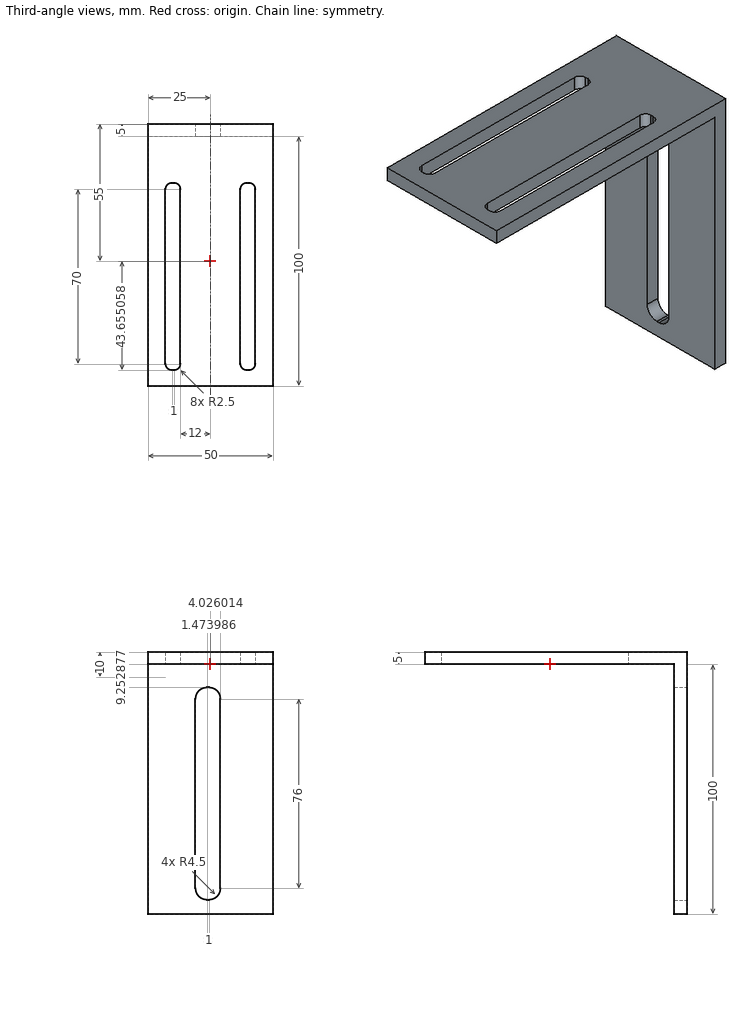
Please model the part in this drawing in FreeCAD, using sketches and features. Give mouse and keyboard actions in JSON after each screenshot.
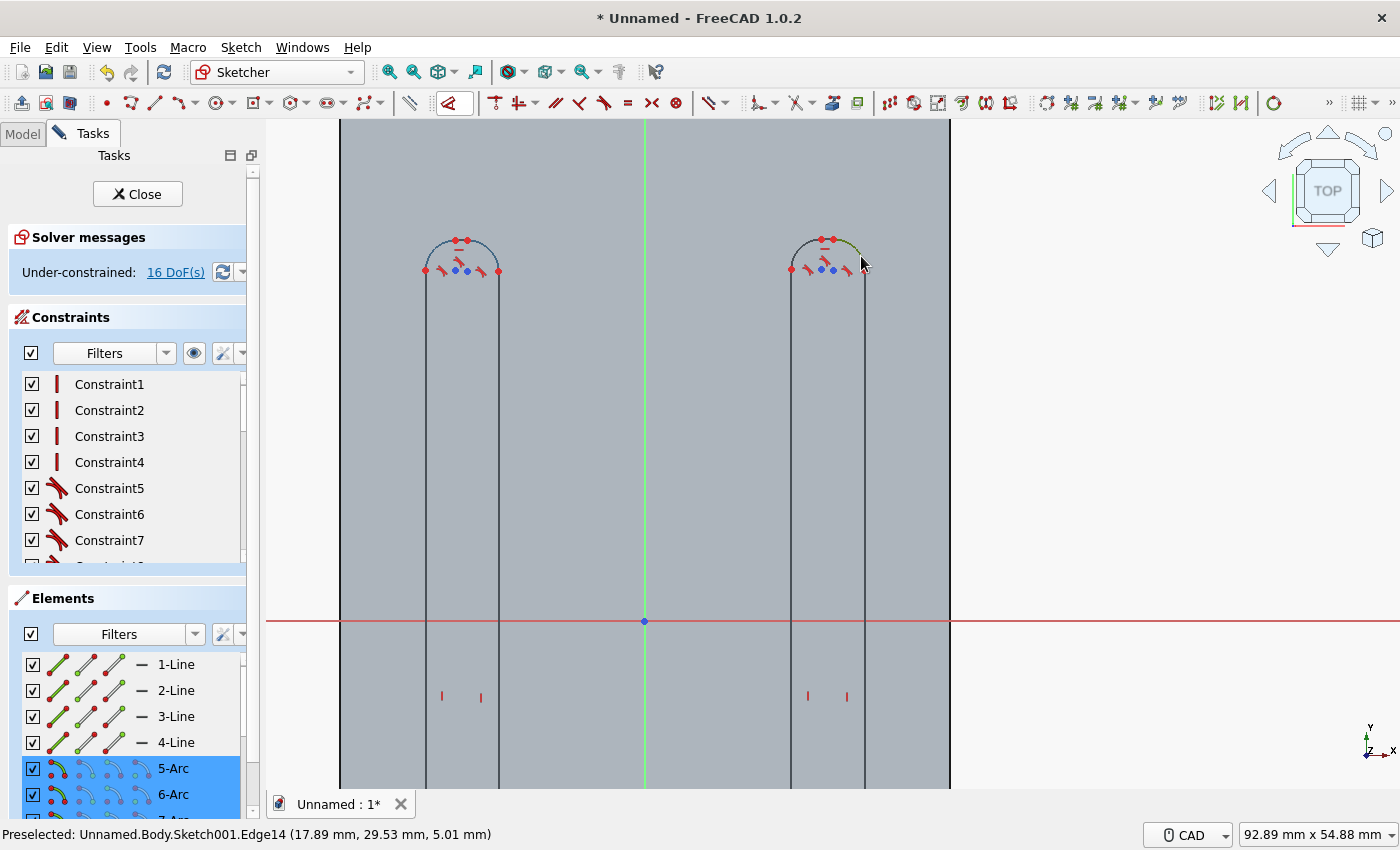
{"action": "left_click", "coordinate": [808, 243]}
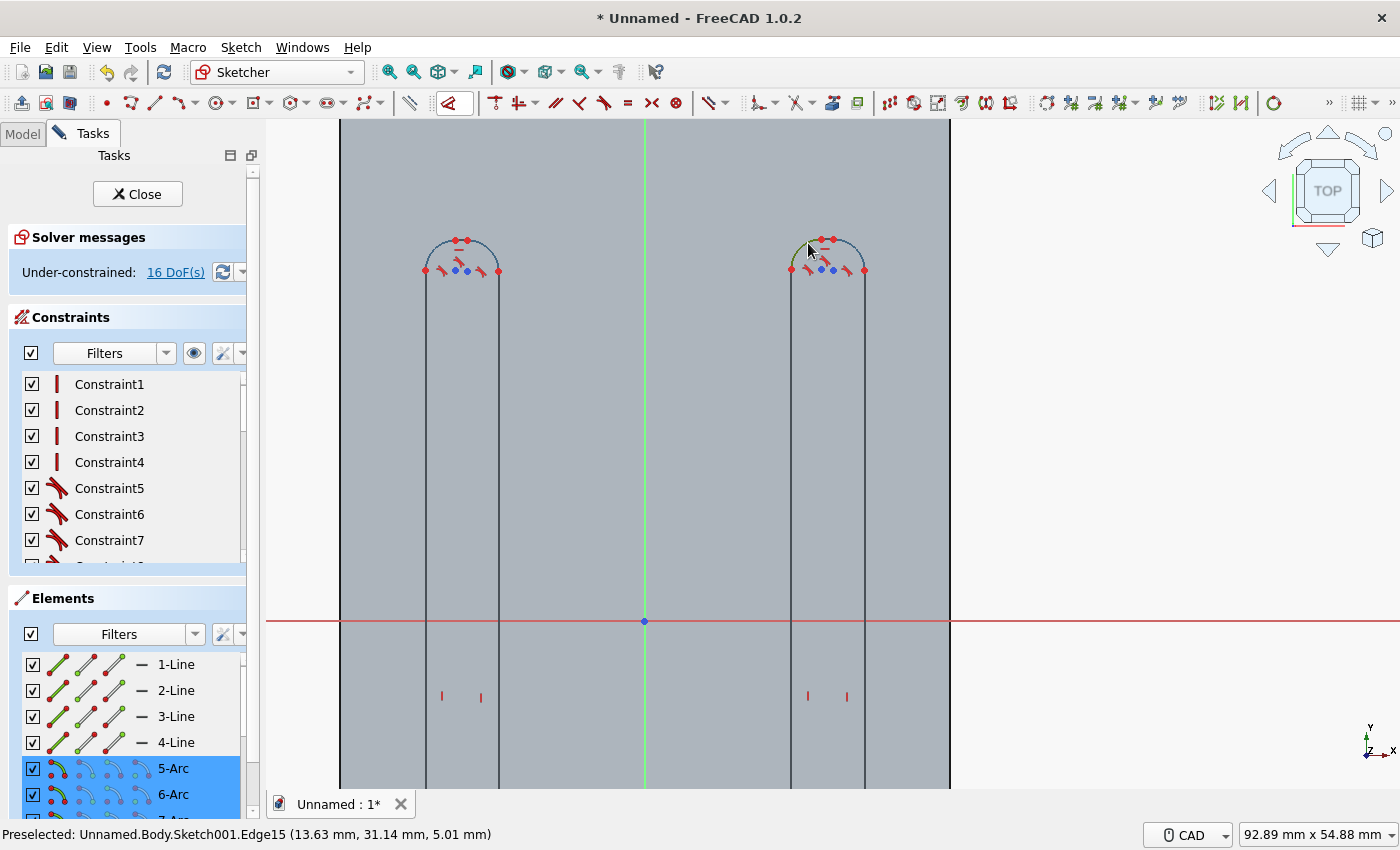
{"action": "scroll", "coordinate": [862, 256], "scroll_direction": "down", "scroll_amount": 4}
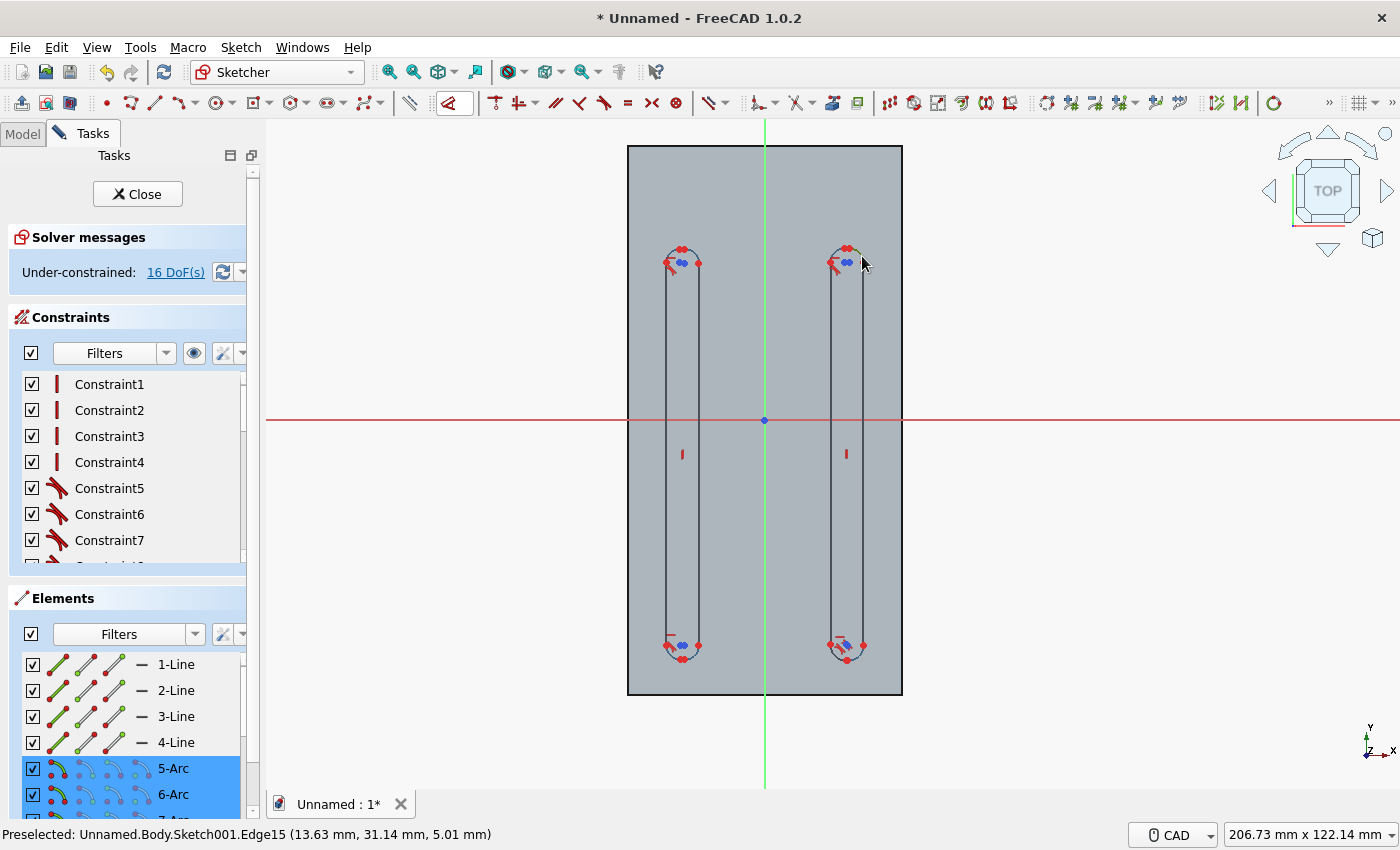
{"action": "scroll", "coordinate": [832, 652], "scroll_direction": "up", "scroll_amount": 4}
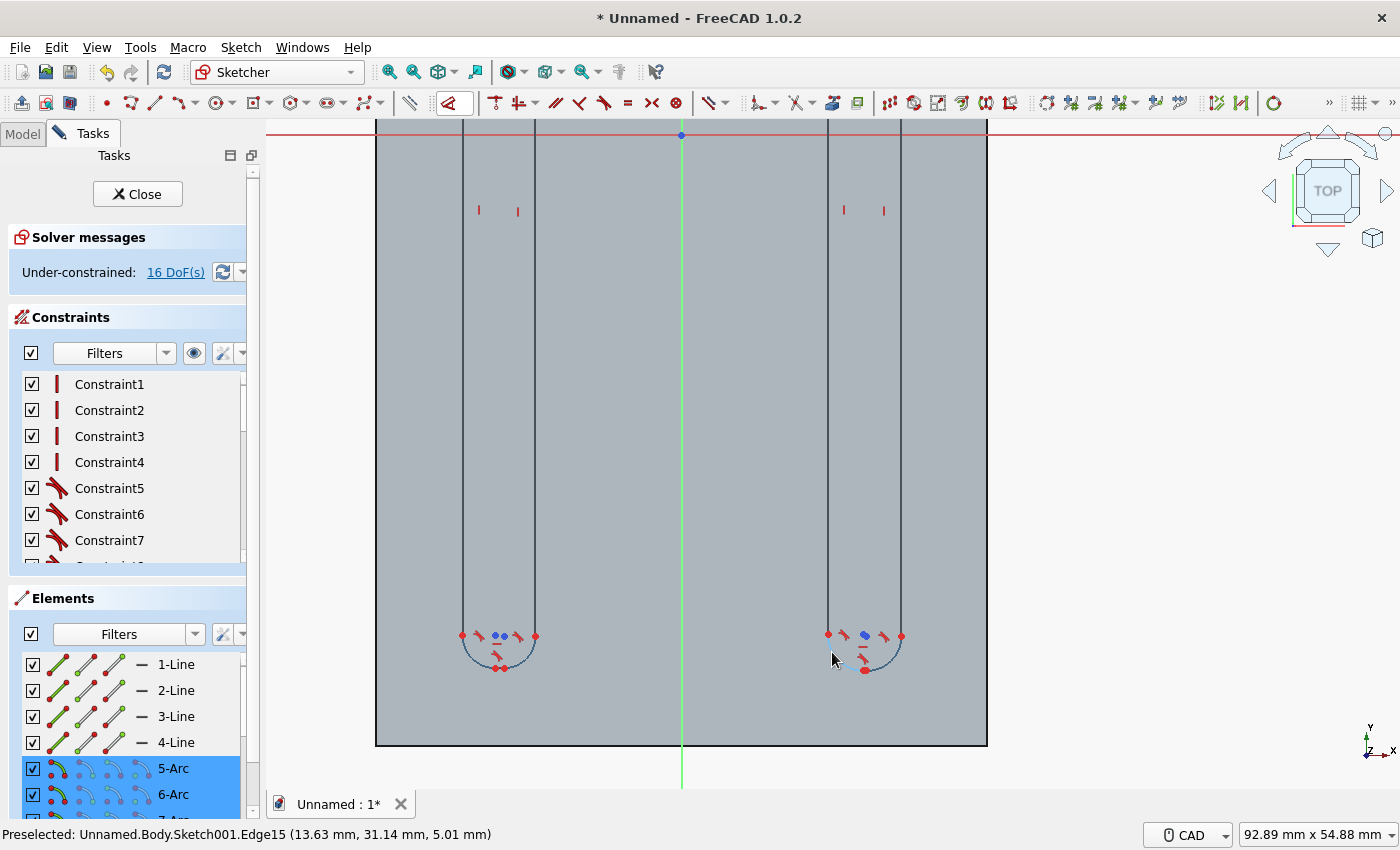
{"action": "left_click", "coordinate": [832, 651]}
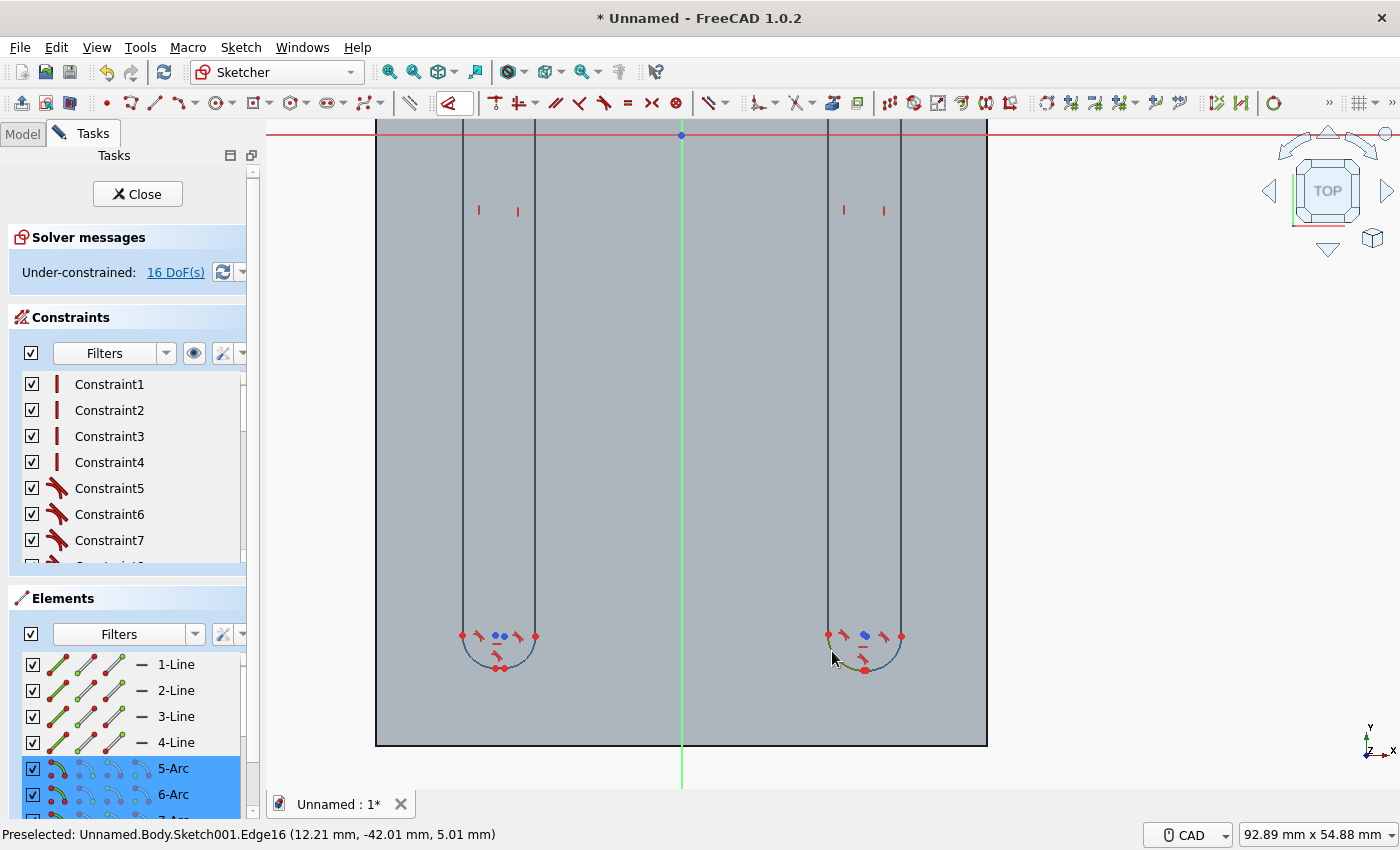
{"action": "left_click", "coordinate": [628, 104]}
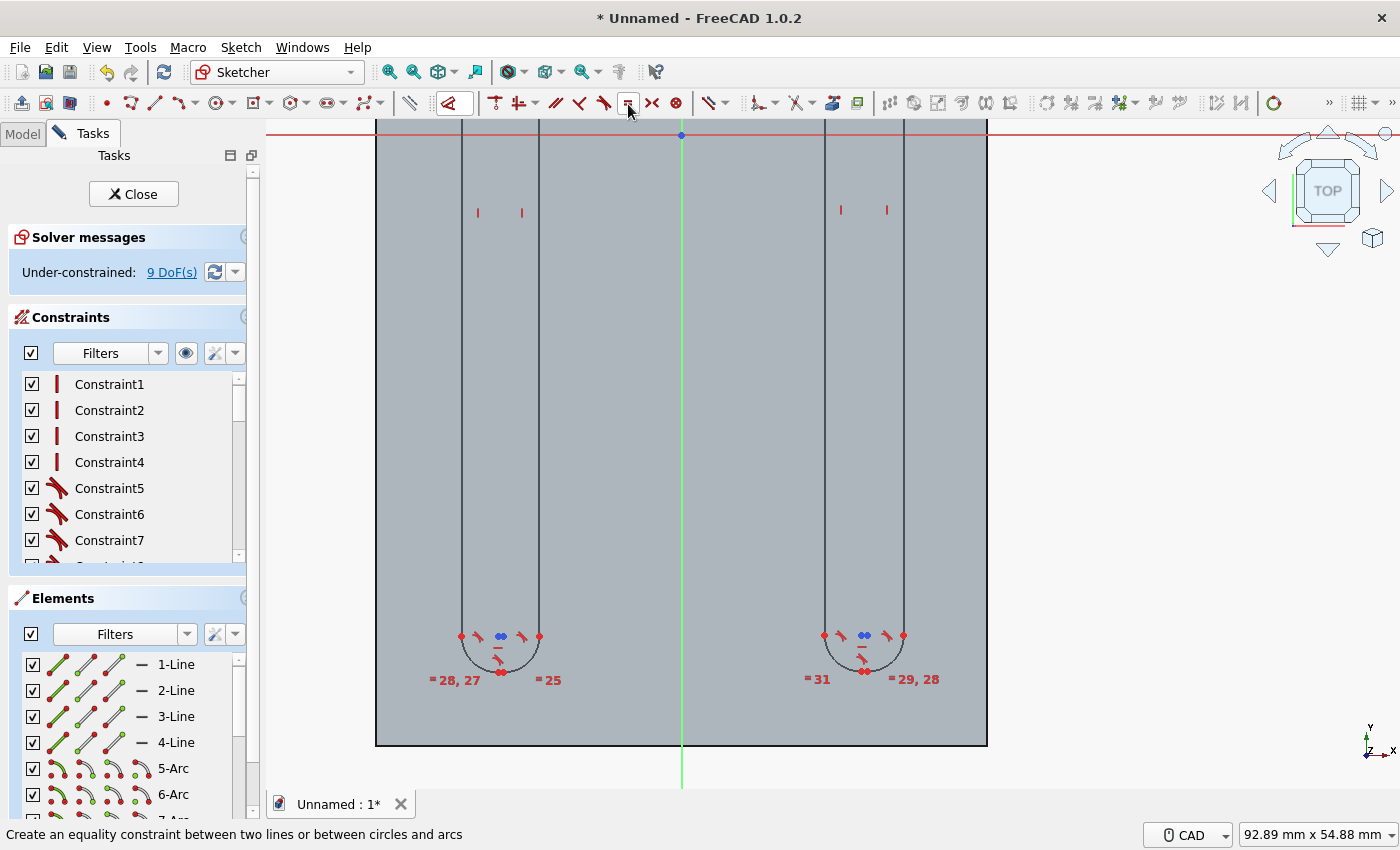
{"action": "scroll", "coordinate": [498, 636], "scroll_direction": "up", "scroll_amount": 5}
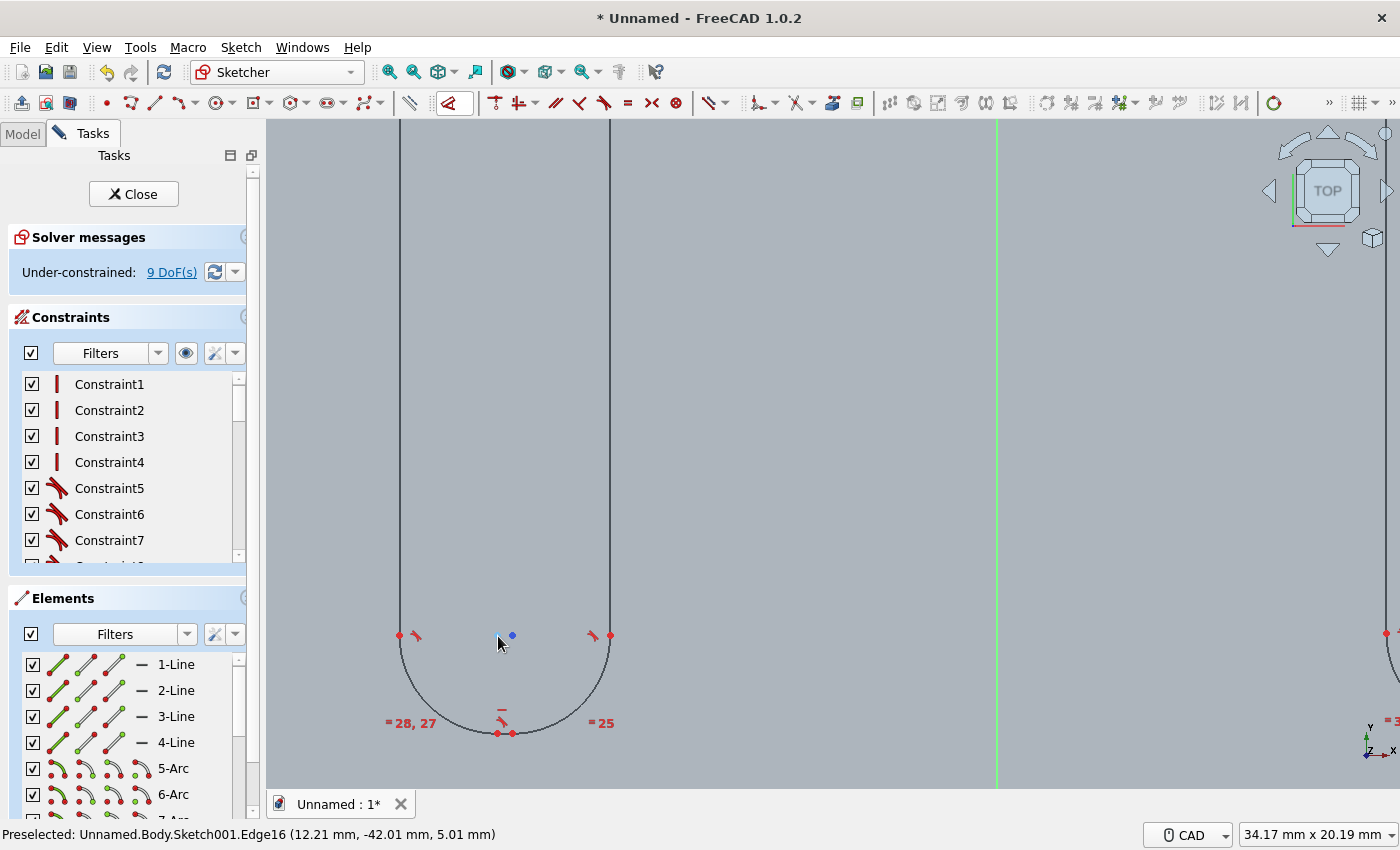
{"action": "left_click", "coordinate": [498, 636]}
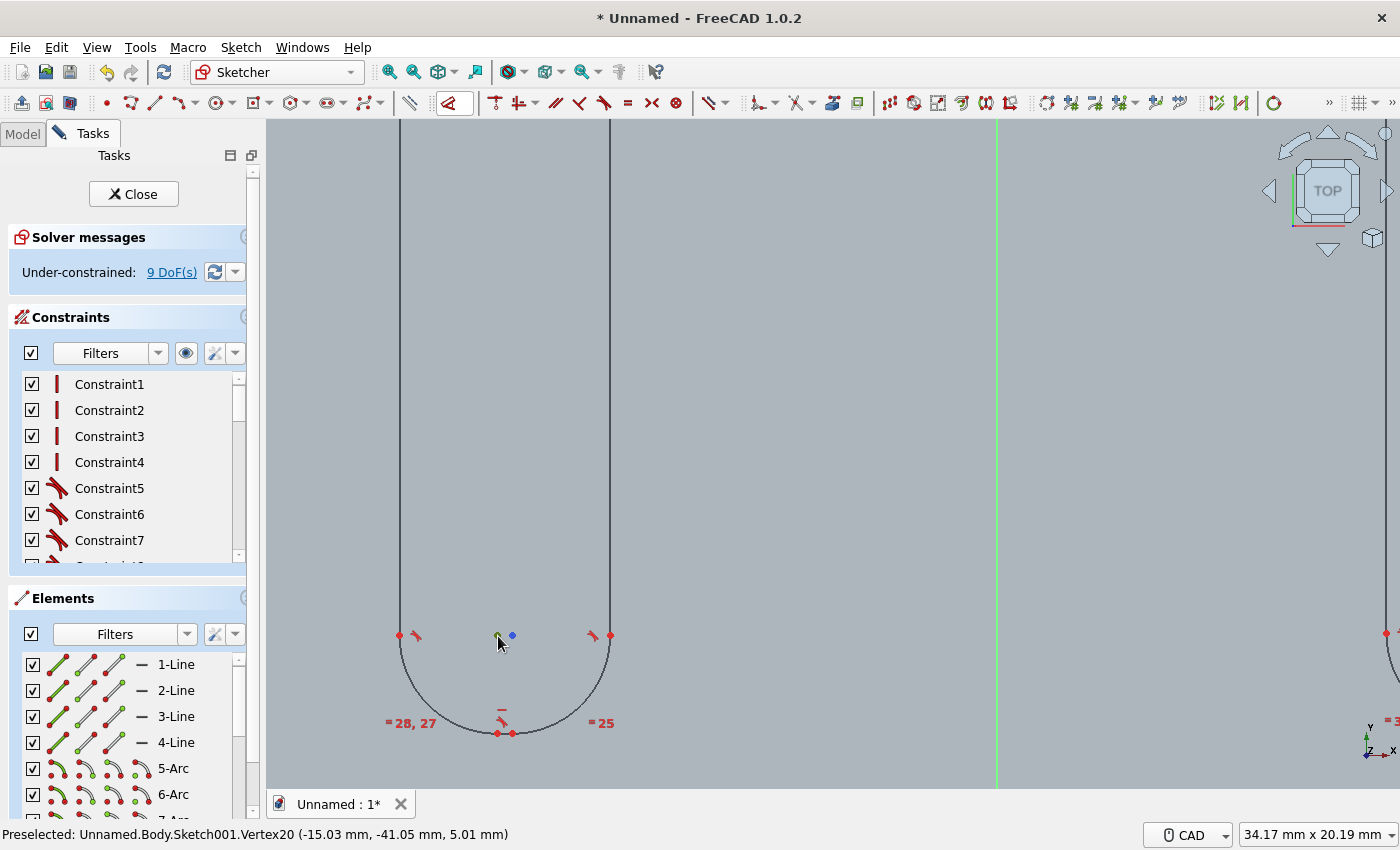
{"action": "scroll", "coordinate": [719, 647], "scroll_direction": "down", "scroll_amount": 9}